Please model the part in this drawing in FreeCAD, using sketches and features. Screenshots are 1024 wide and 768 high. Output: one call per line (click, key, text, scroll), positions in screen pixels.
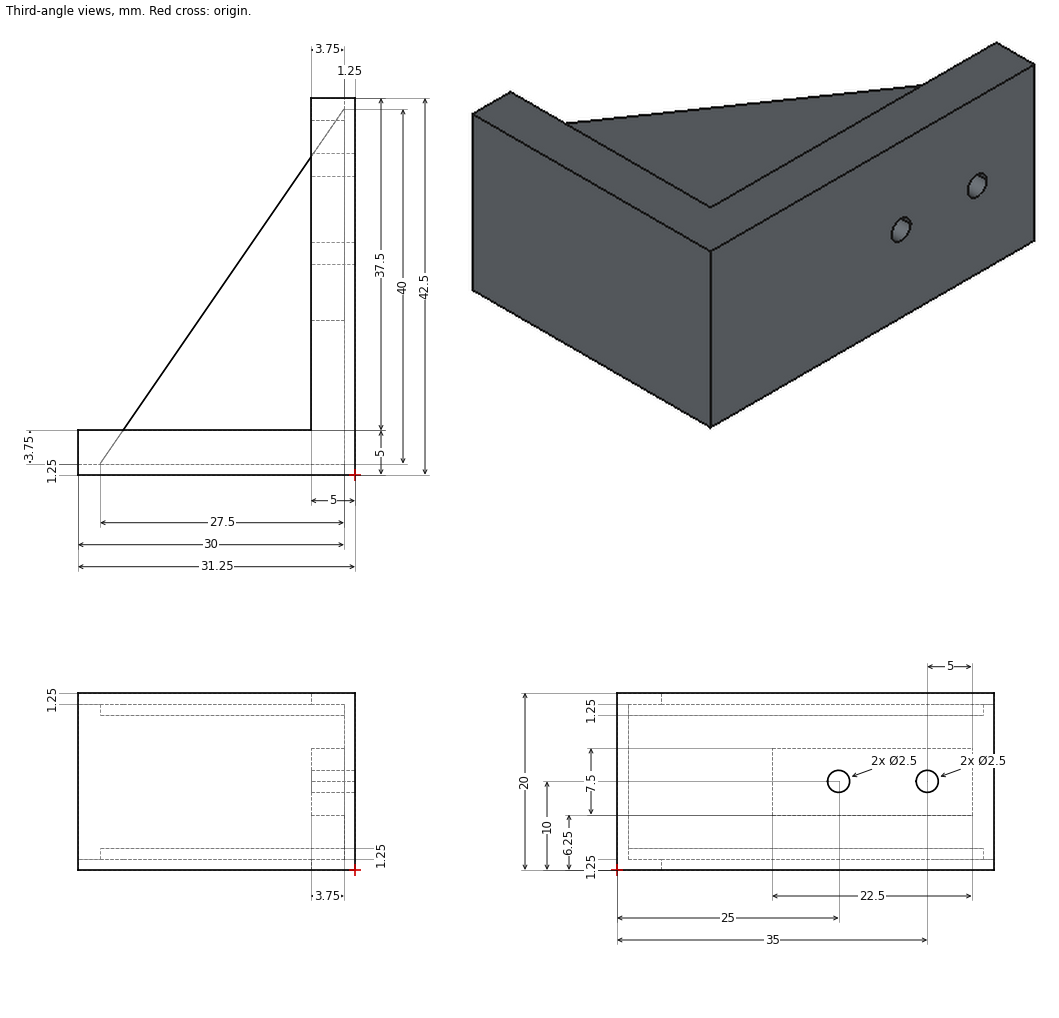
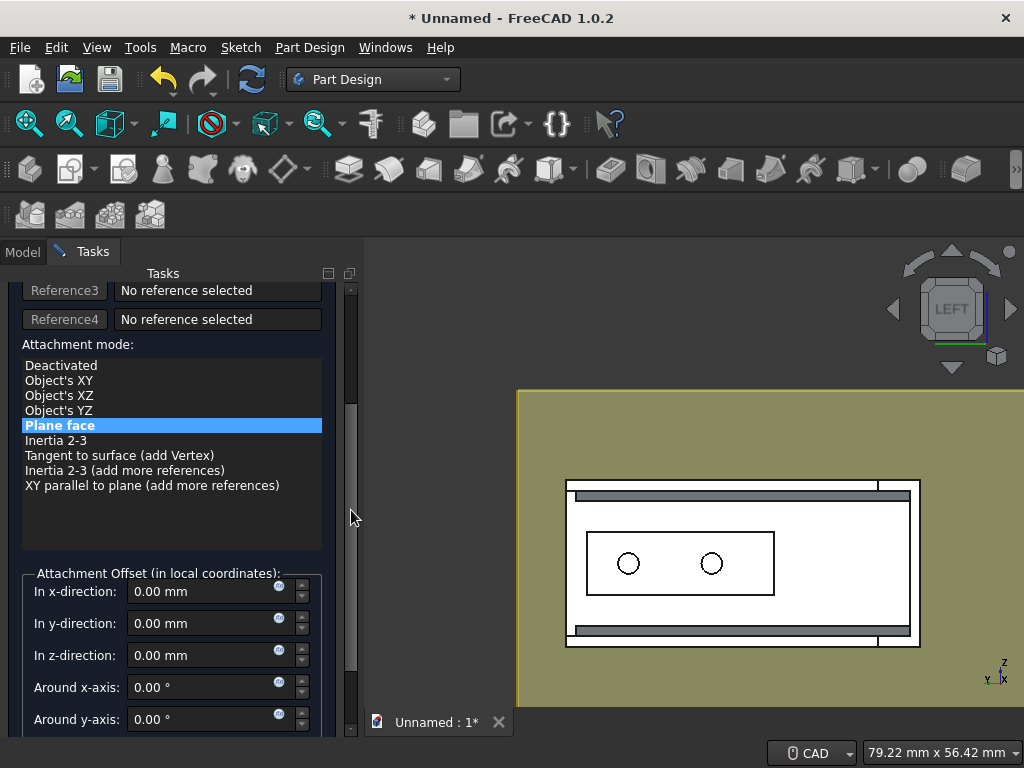
triple_click(210, 655)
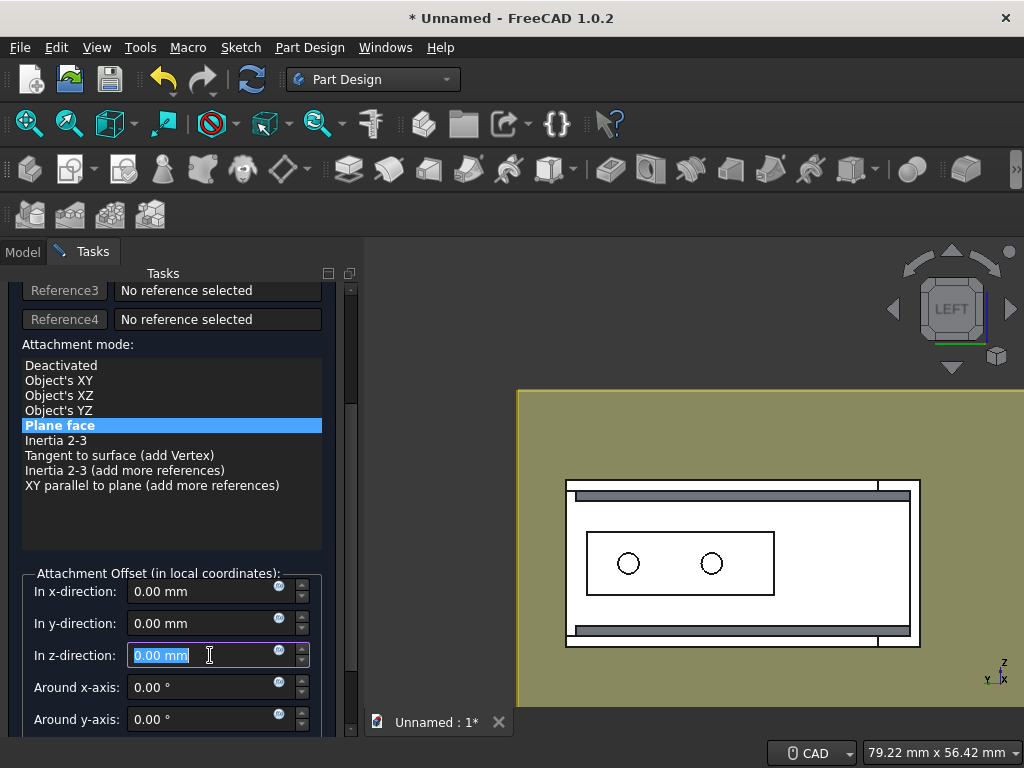
text(2.5)
key(Tab)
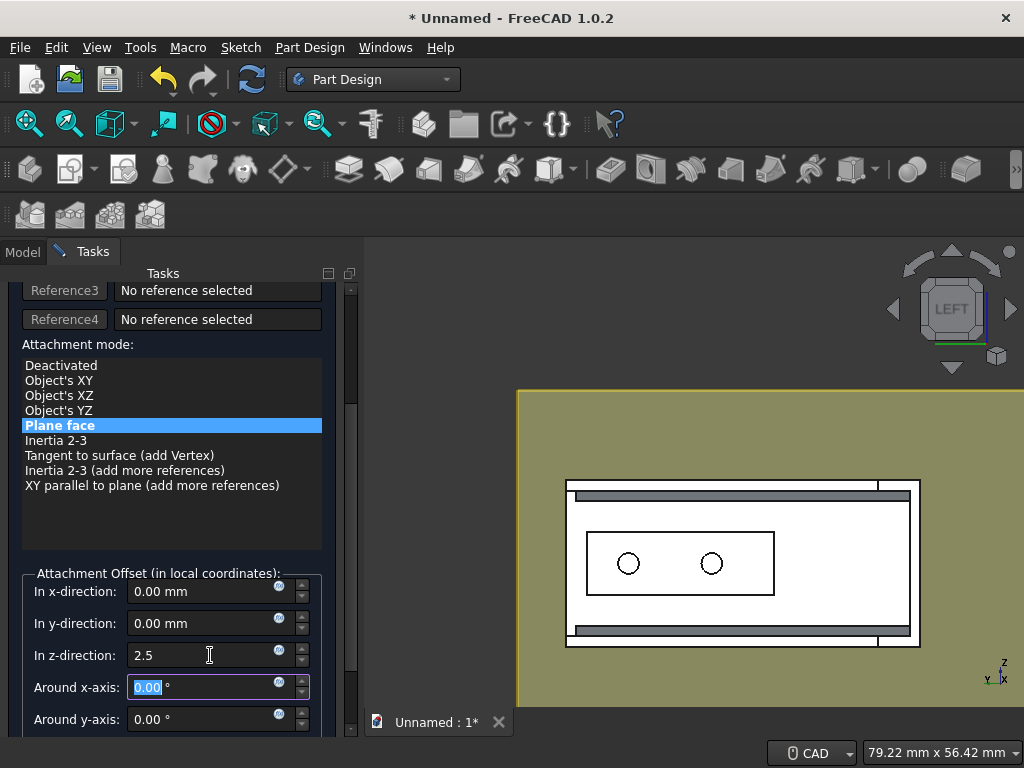
scroll(351, 510, up, 4)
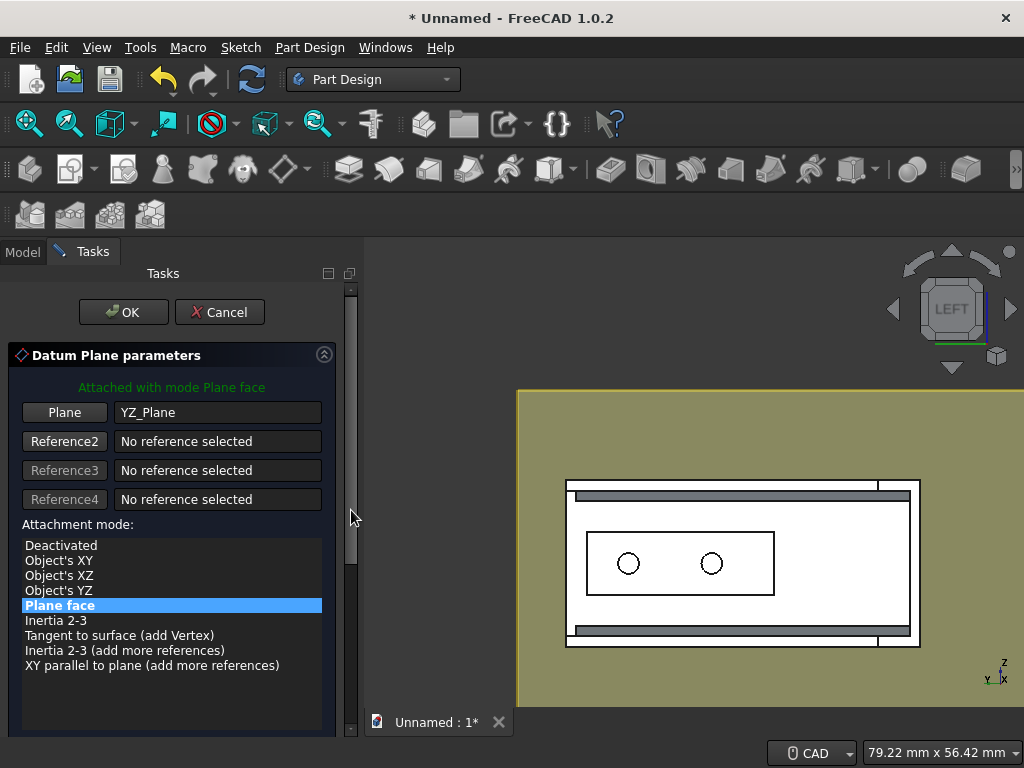
click(124, 312)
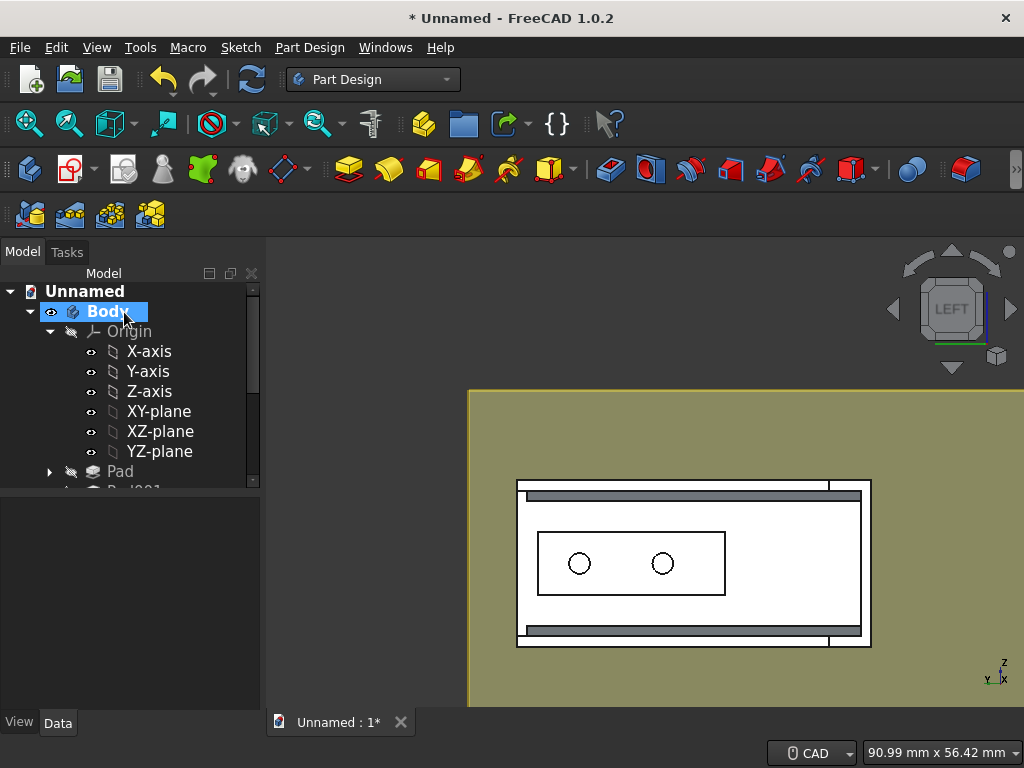
scroll(100, 387, down, 3)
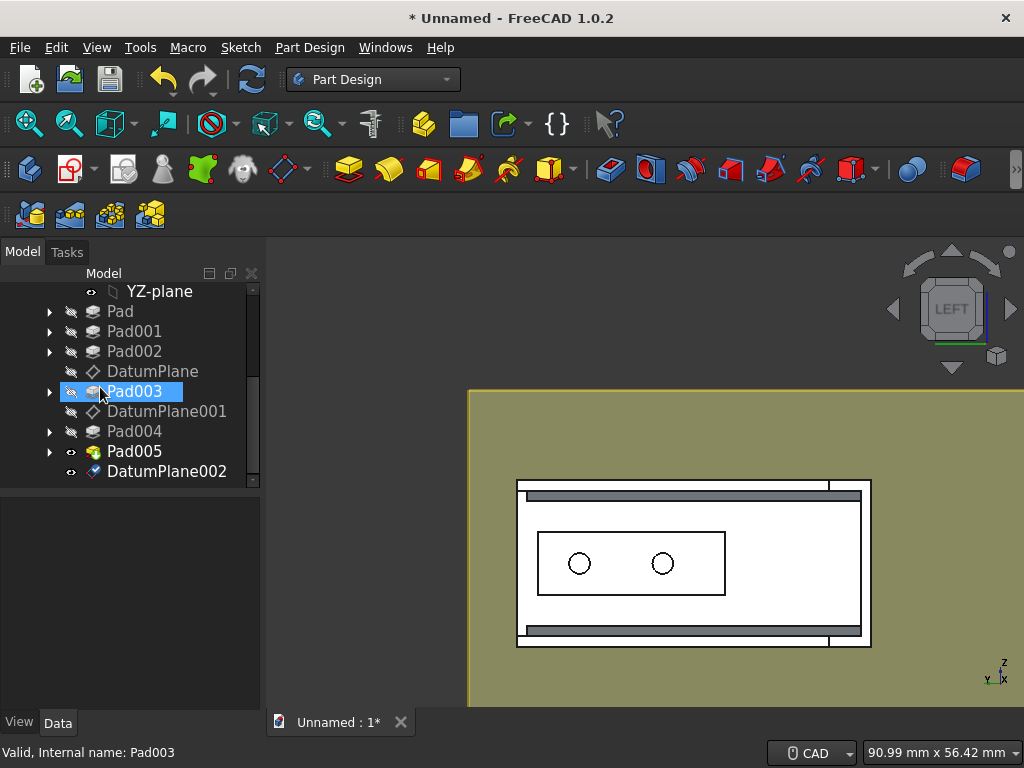
click(116, 472)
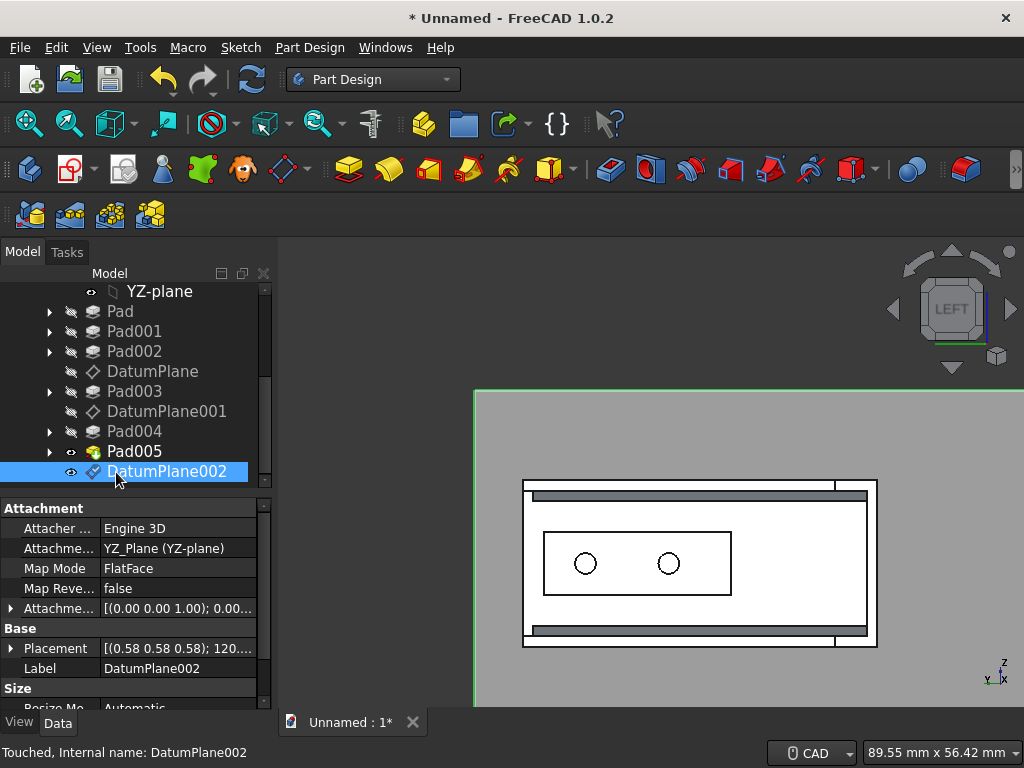
click(70, 170)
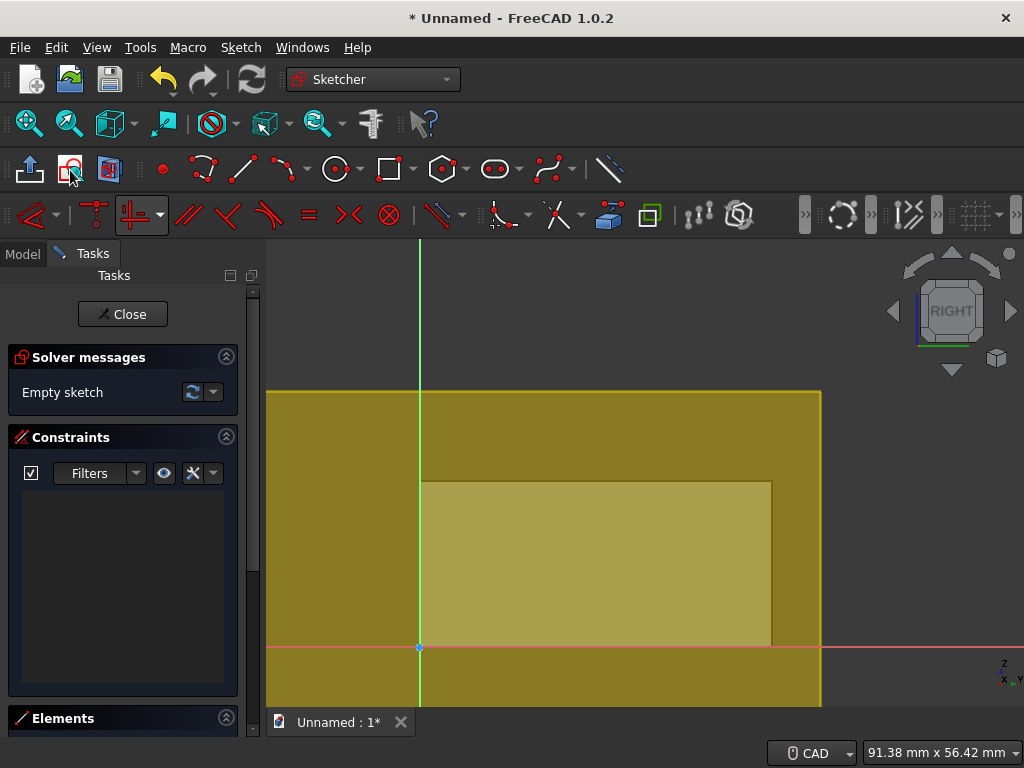
scroll(699, 594, up, 7)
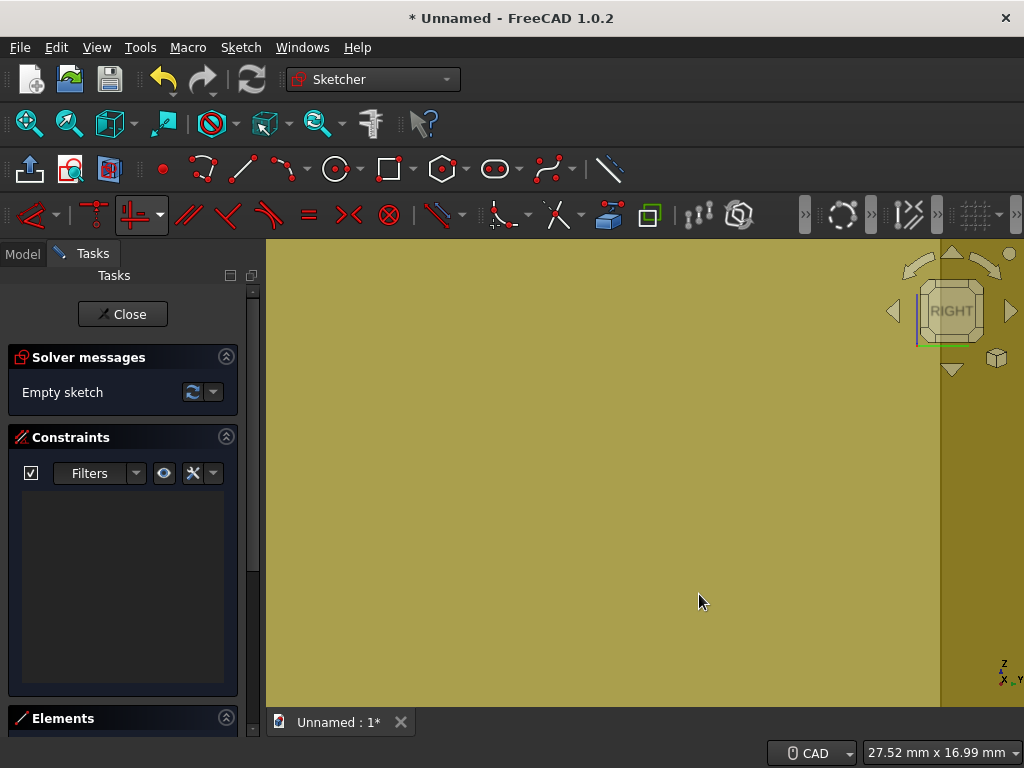
click(336, 170)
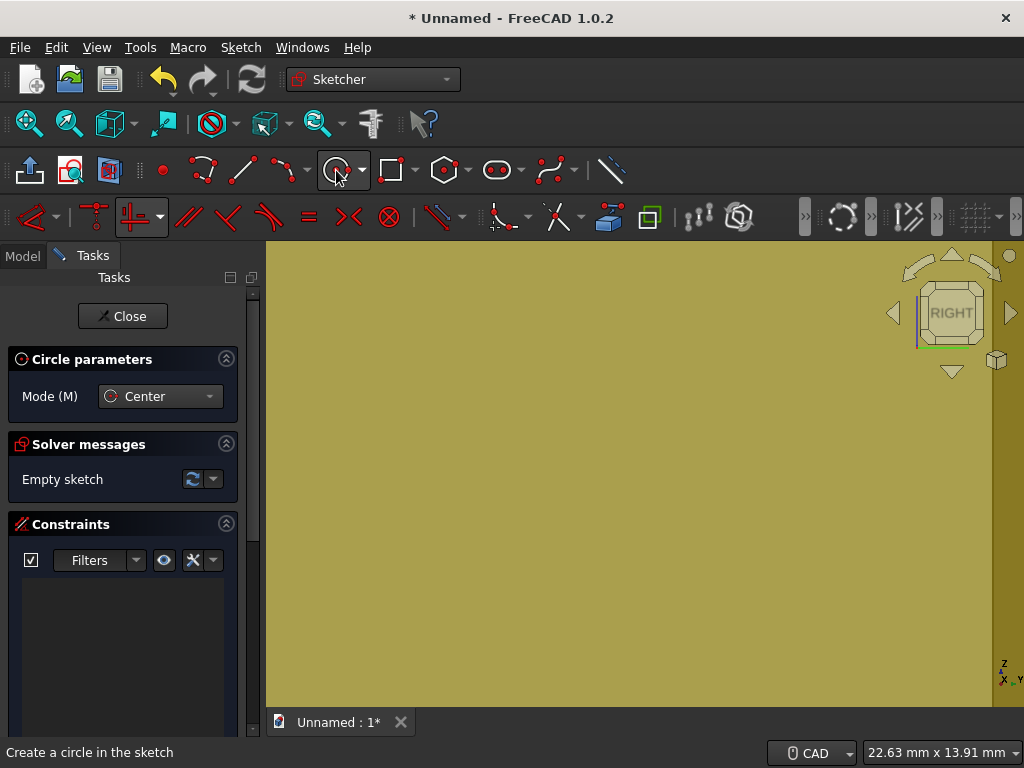
click(742, 471)
move(772, 442)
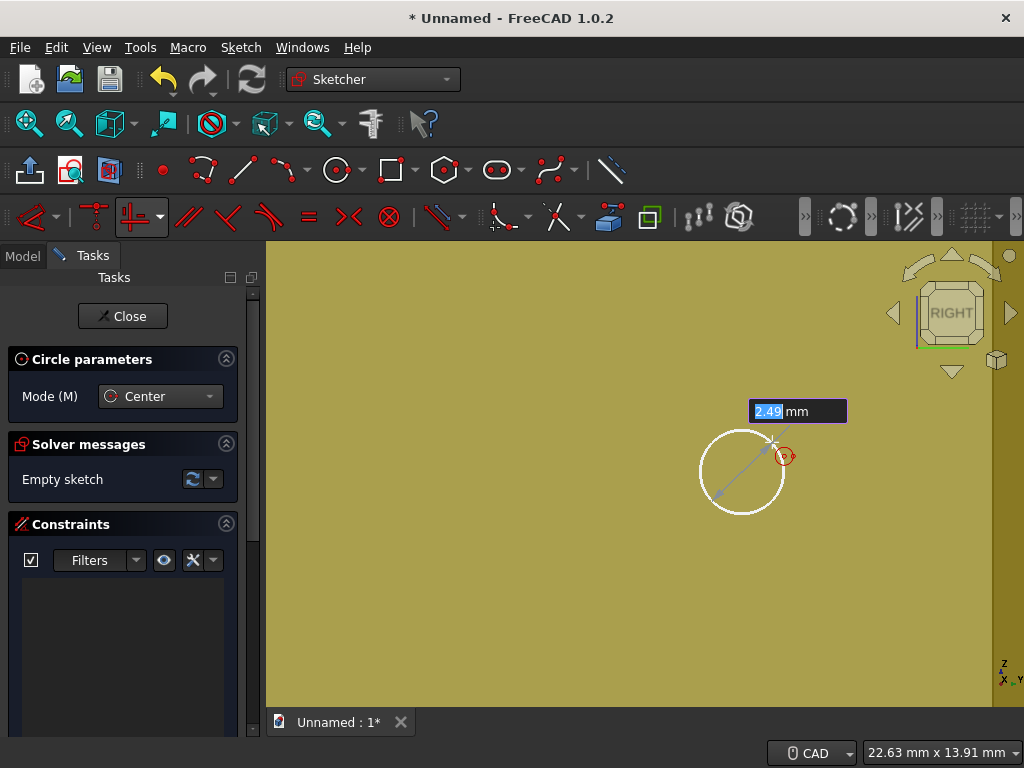
text(2.5)
key(Return)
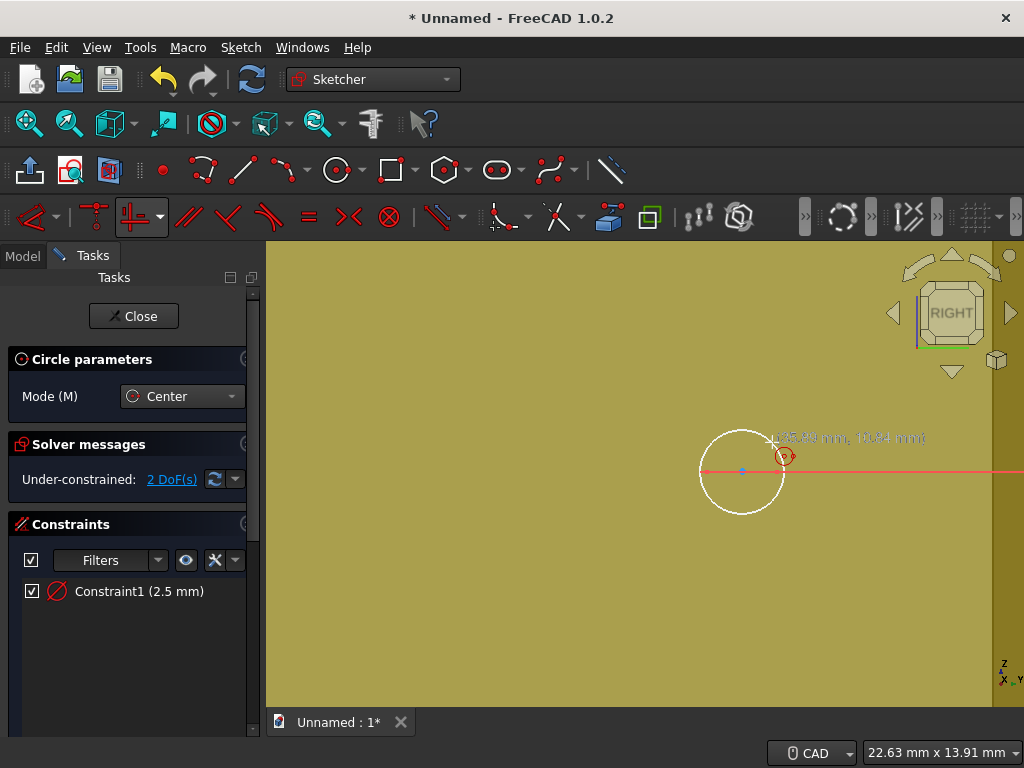
click(407, 471)
move(437, 442)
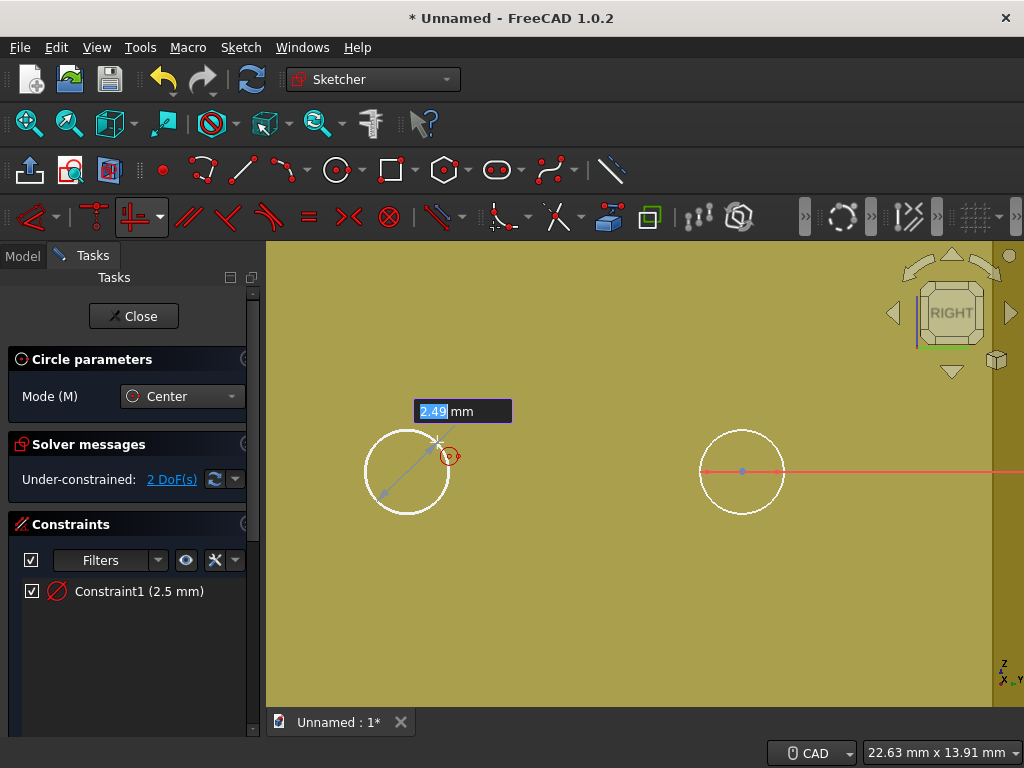
text(2.5)
key(Return)
key(Escape)